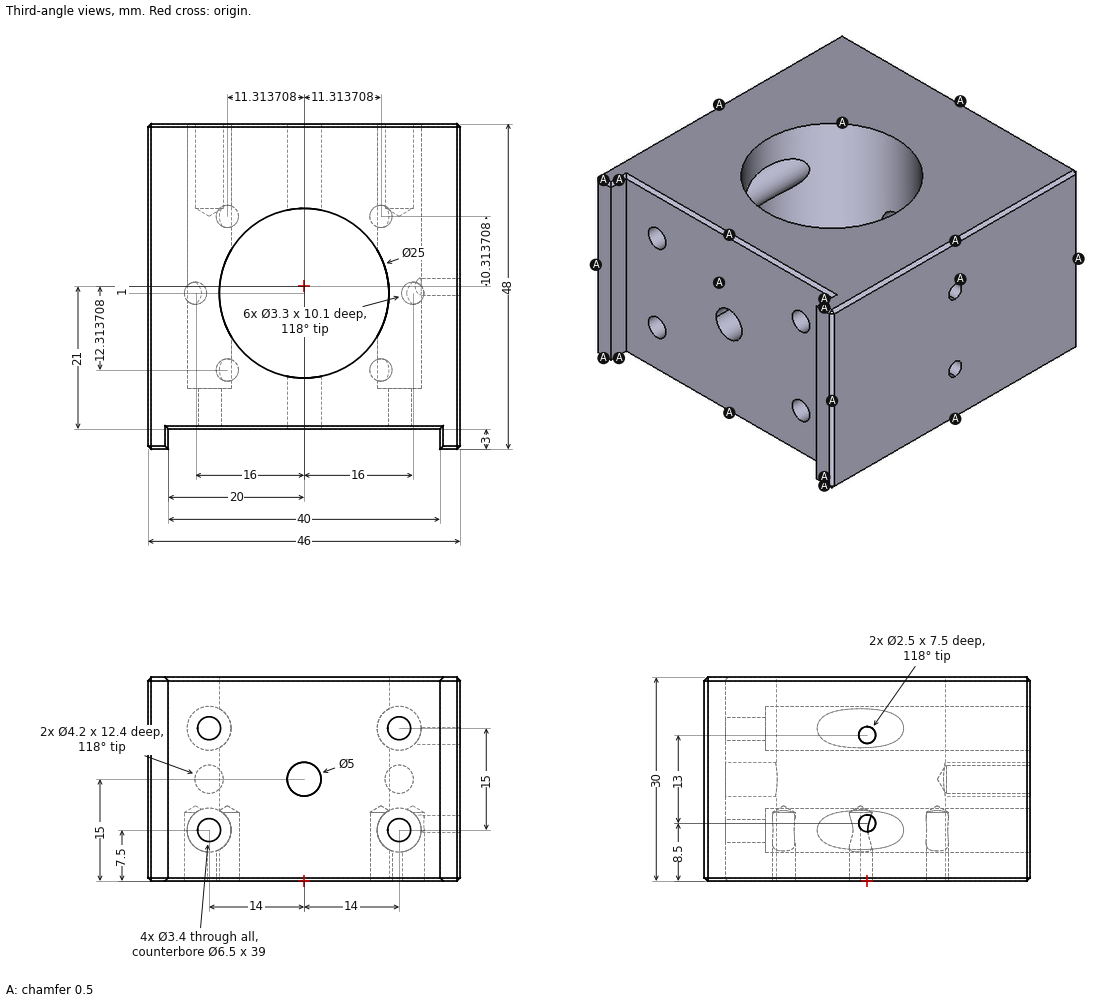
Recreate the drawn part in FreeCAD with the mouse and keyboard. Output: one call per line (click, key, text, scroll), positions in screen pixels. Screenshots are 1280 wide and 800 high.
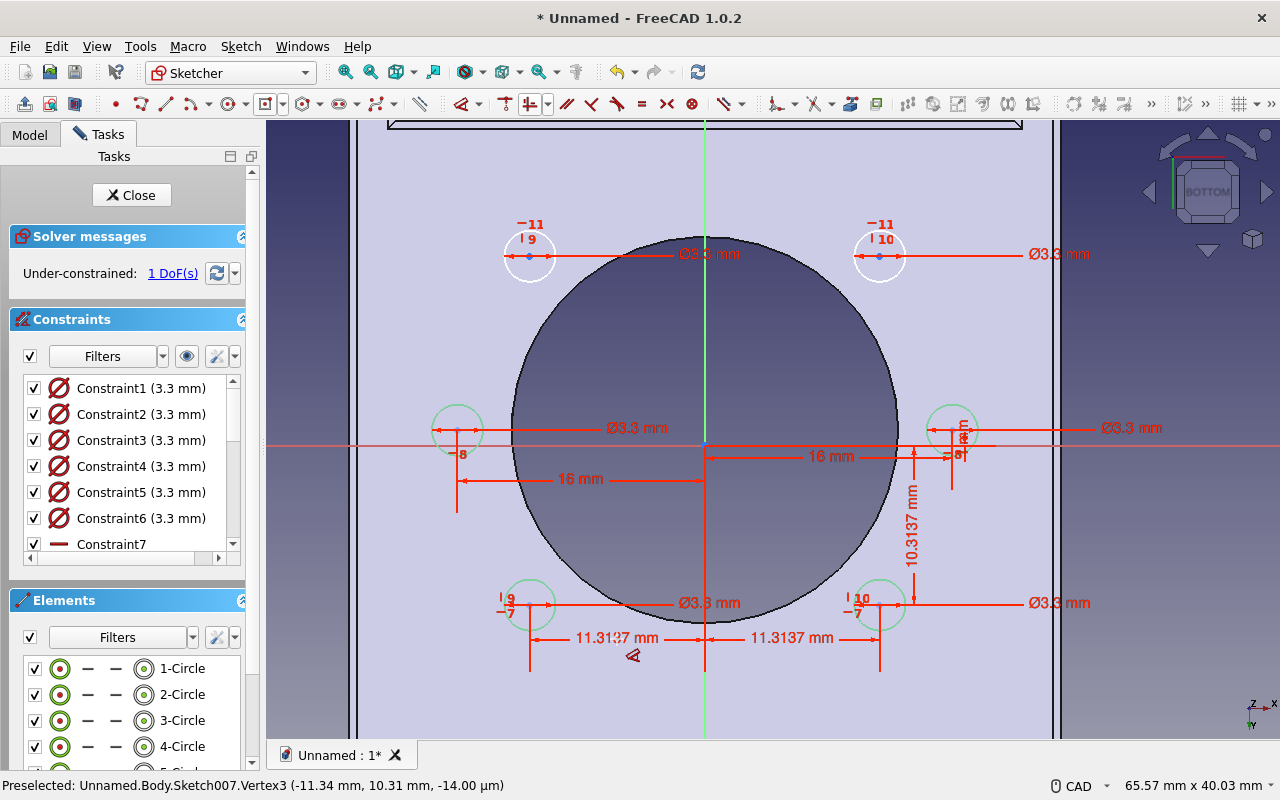
click(530, 256)
click(496, 351)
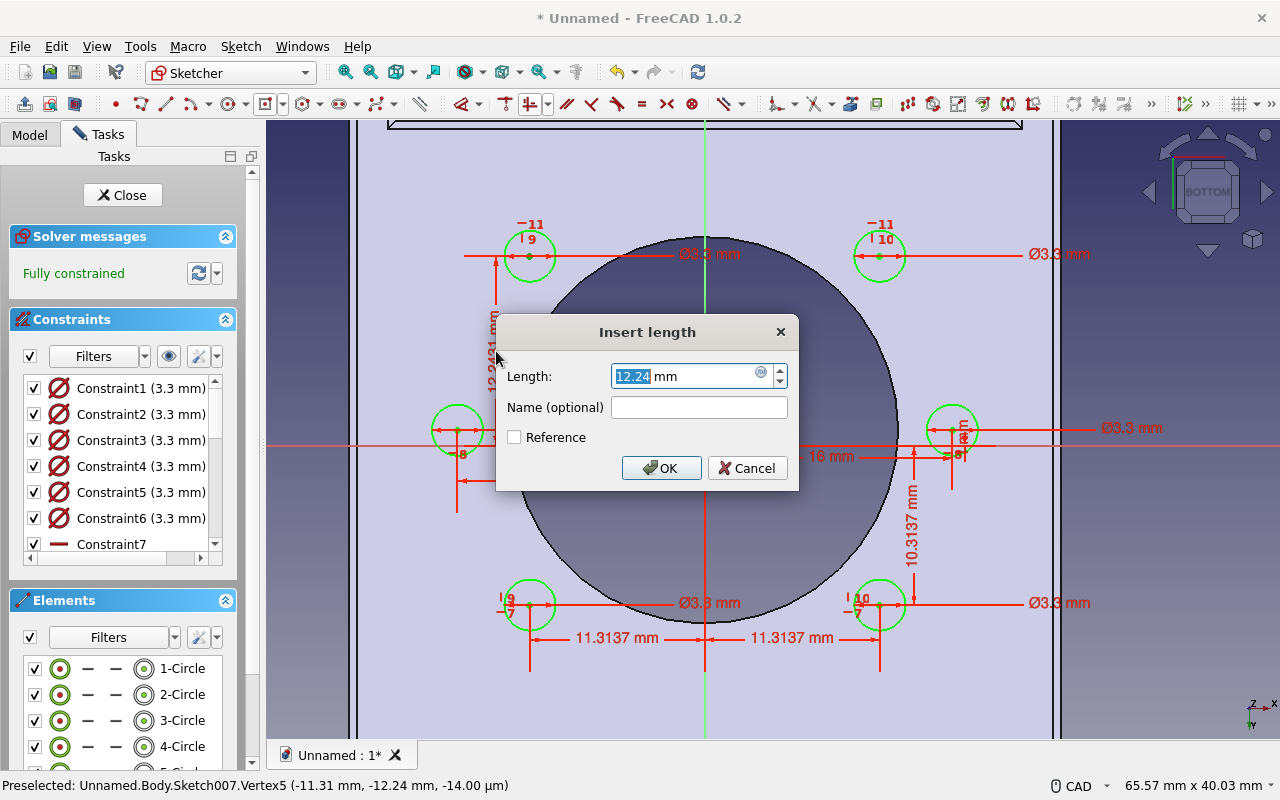
text(12.313708)
key(Return)
key(Escape)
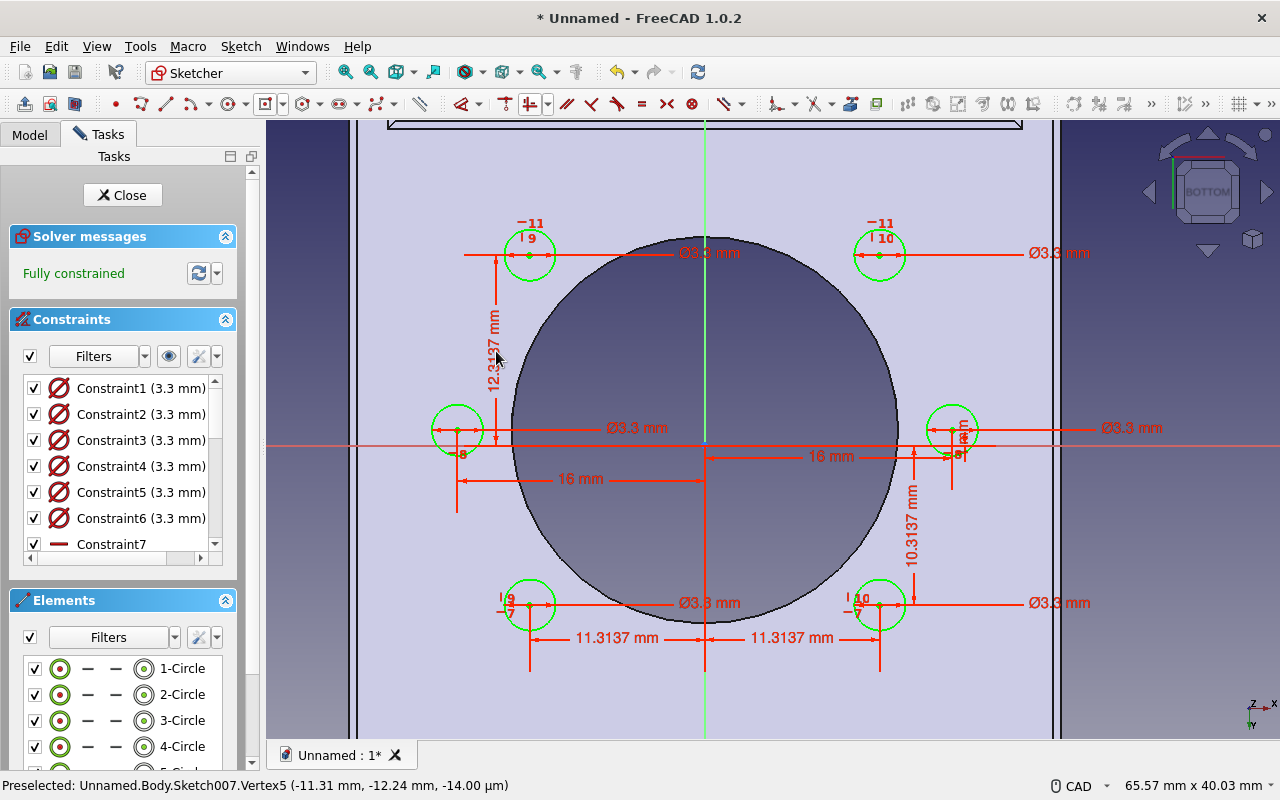
click(123, 195)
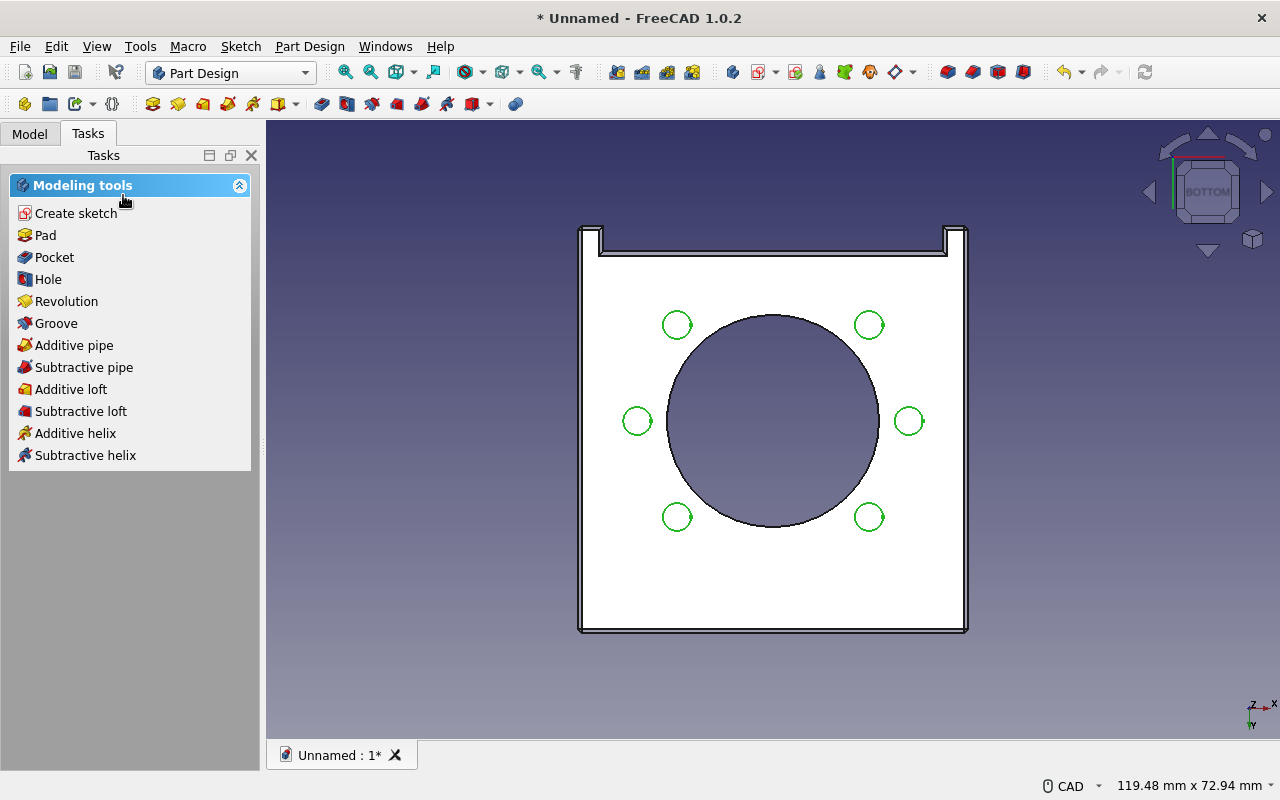
click(347, 104)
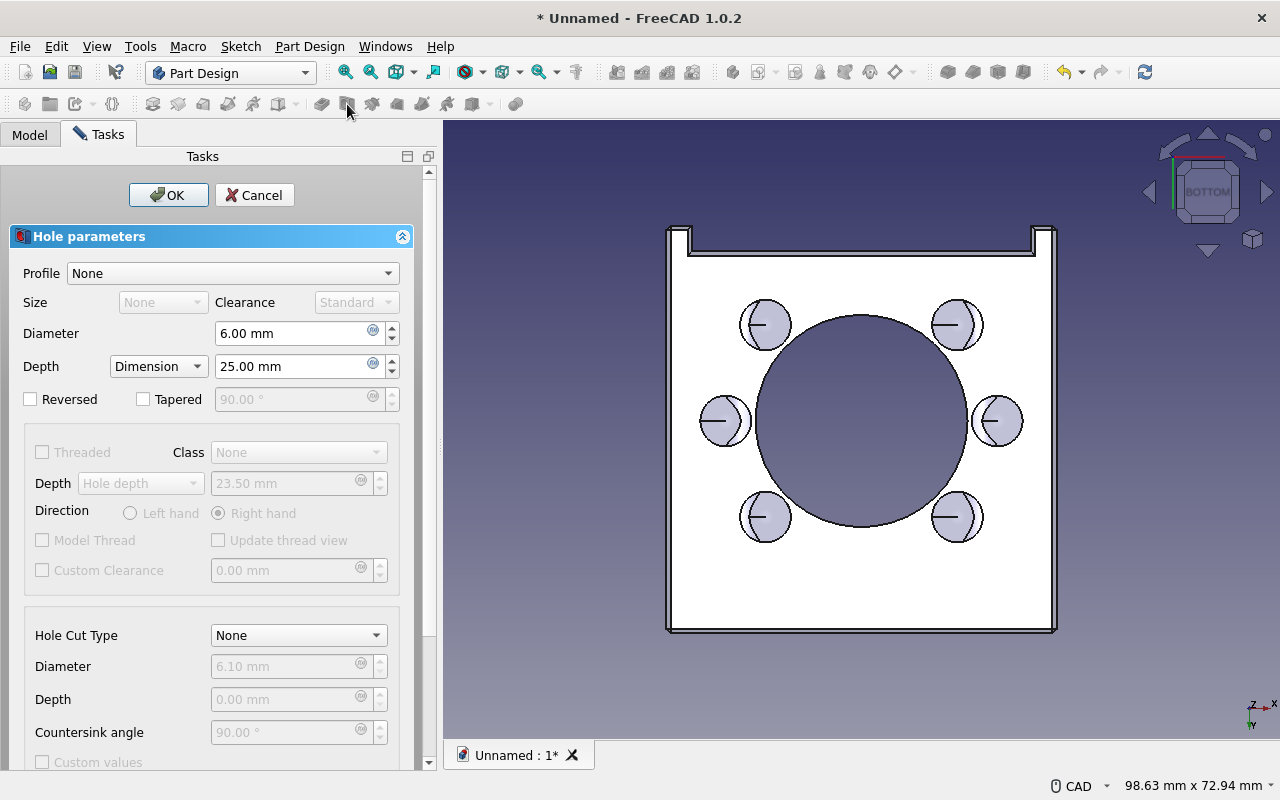
triple_click(300, 334)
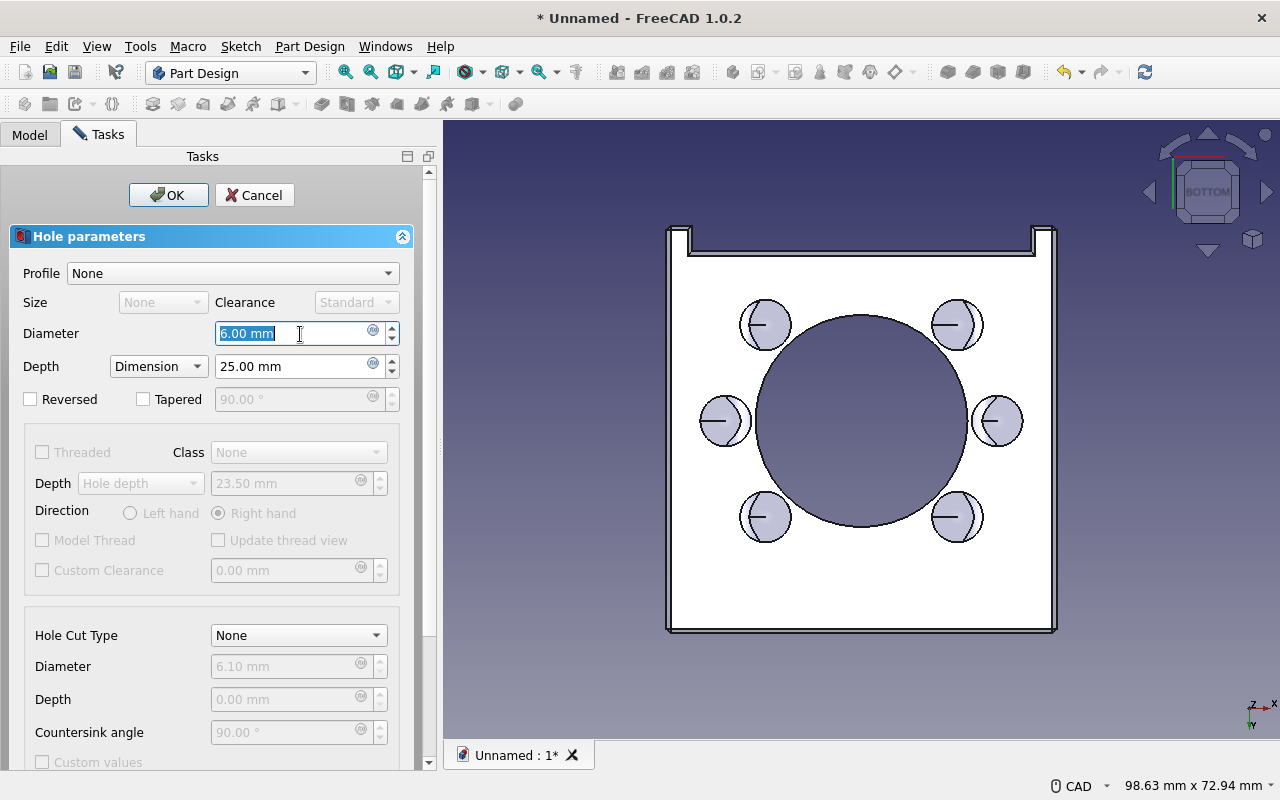
text(3.3)
key(Tab)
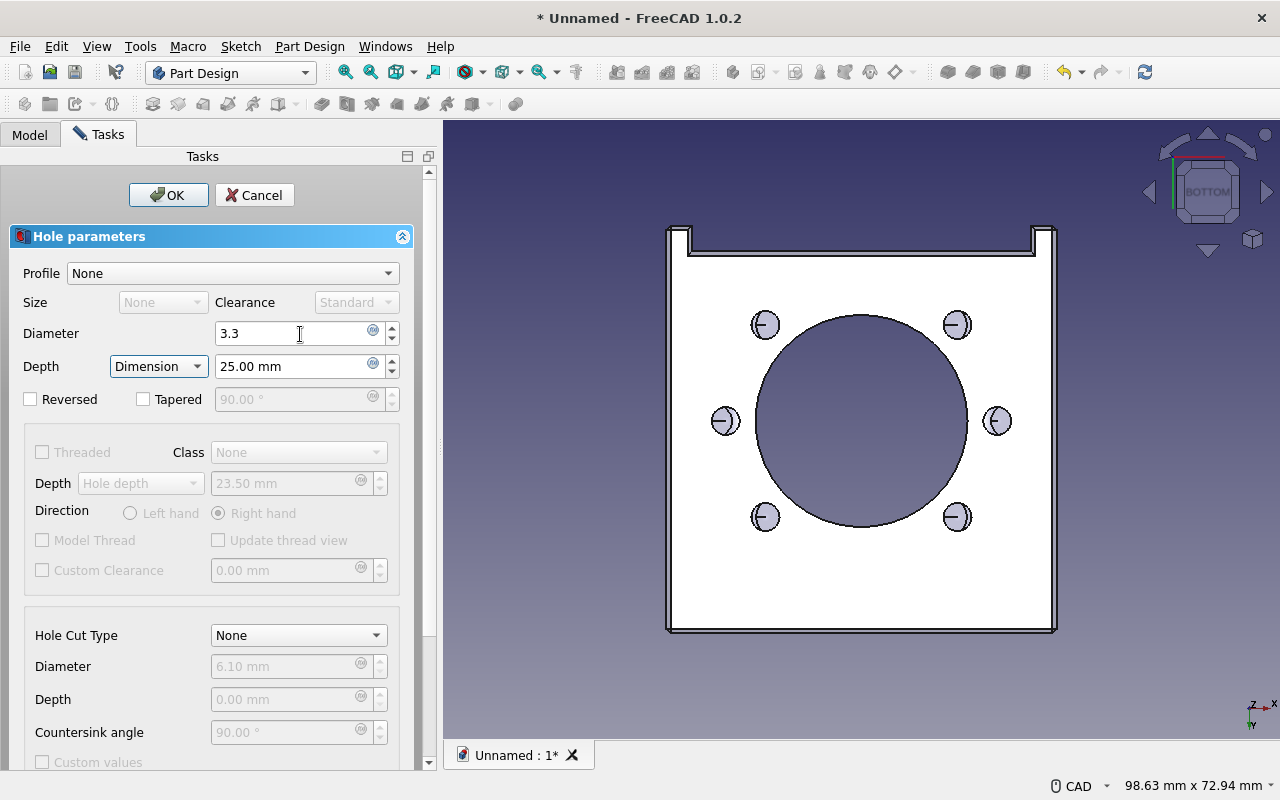
triple_click(300, 366)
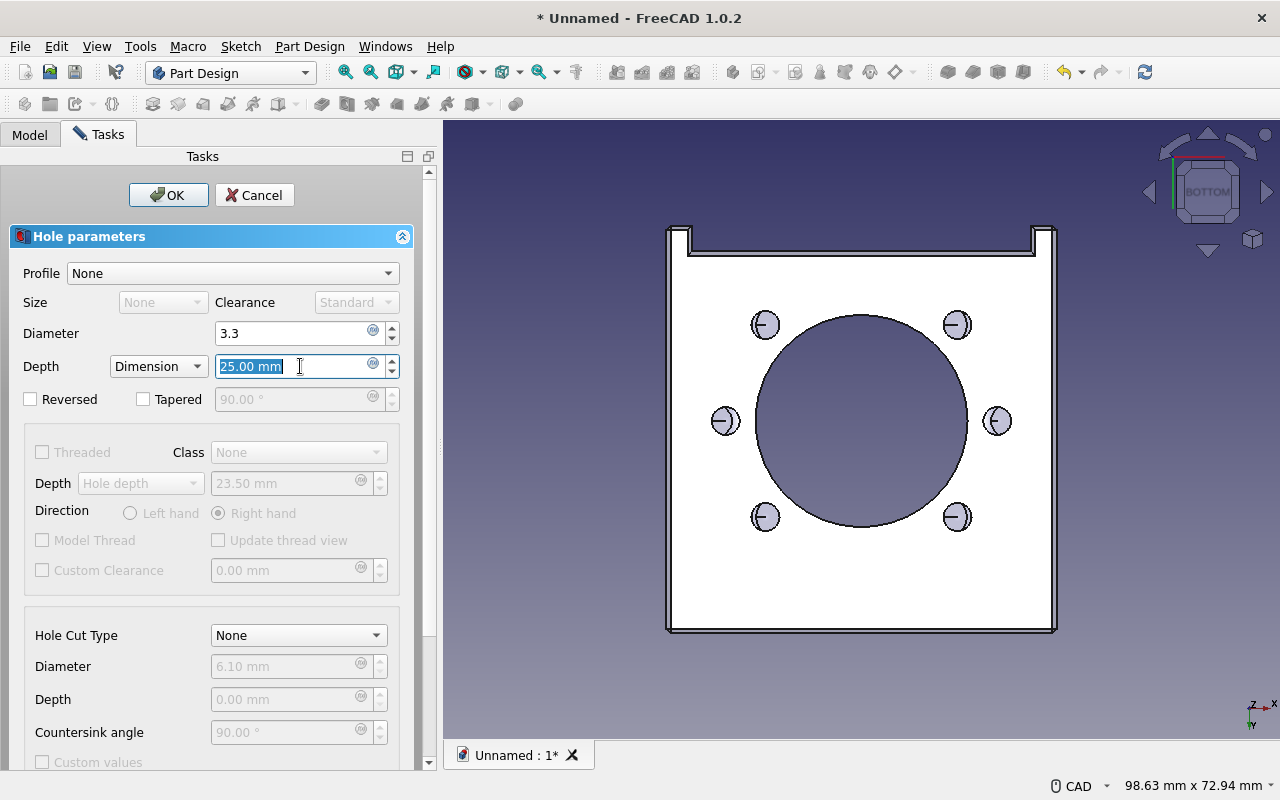
text(10.1)
key(Tab)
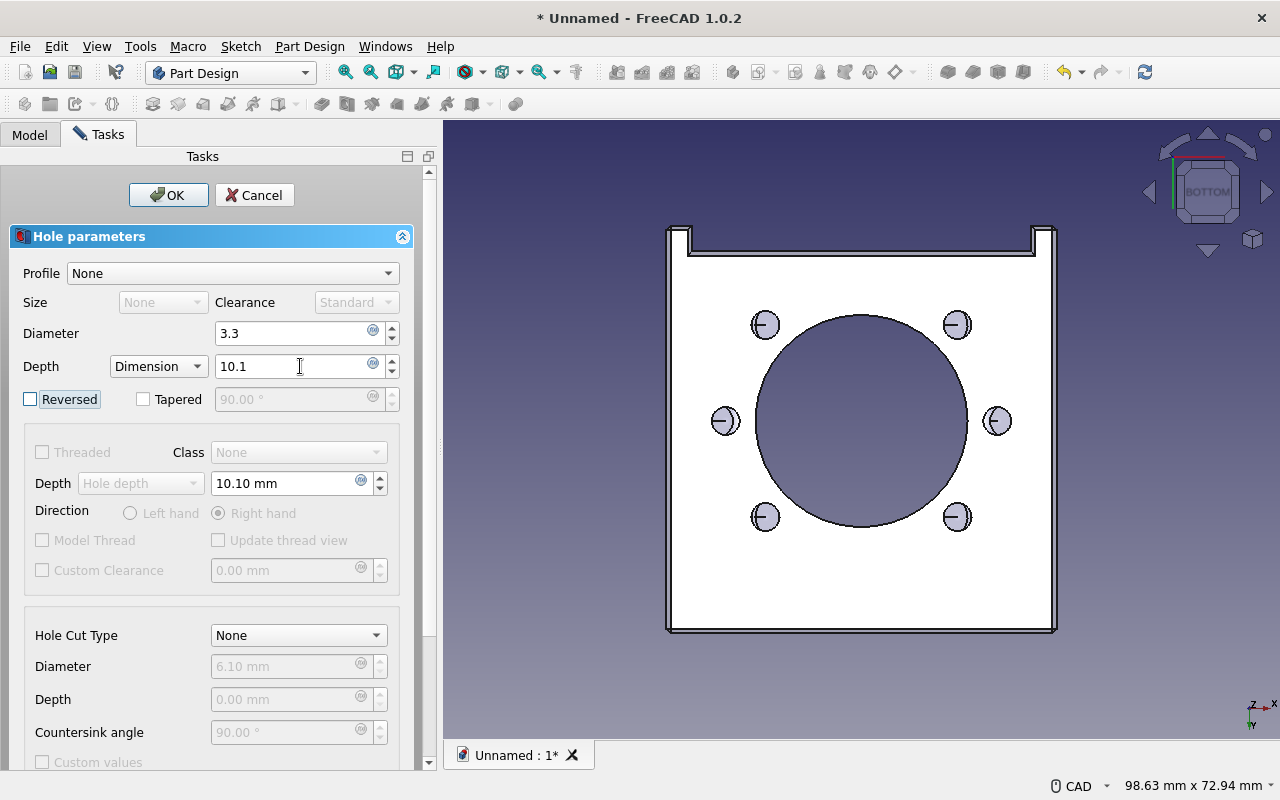
click(169, 195)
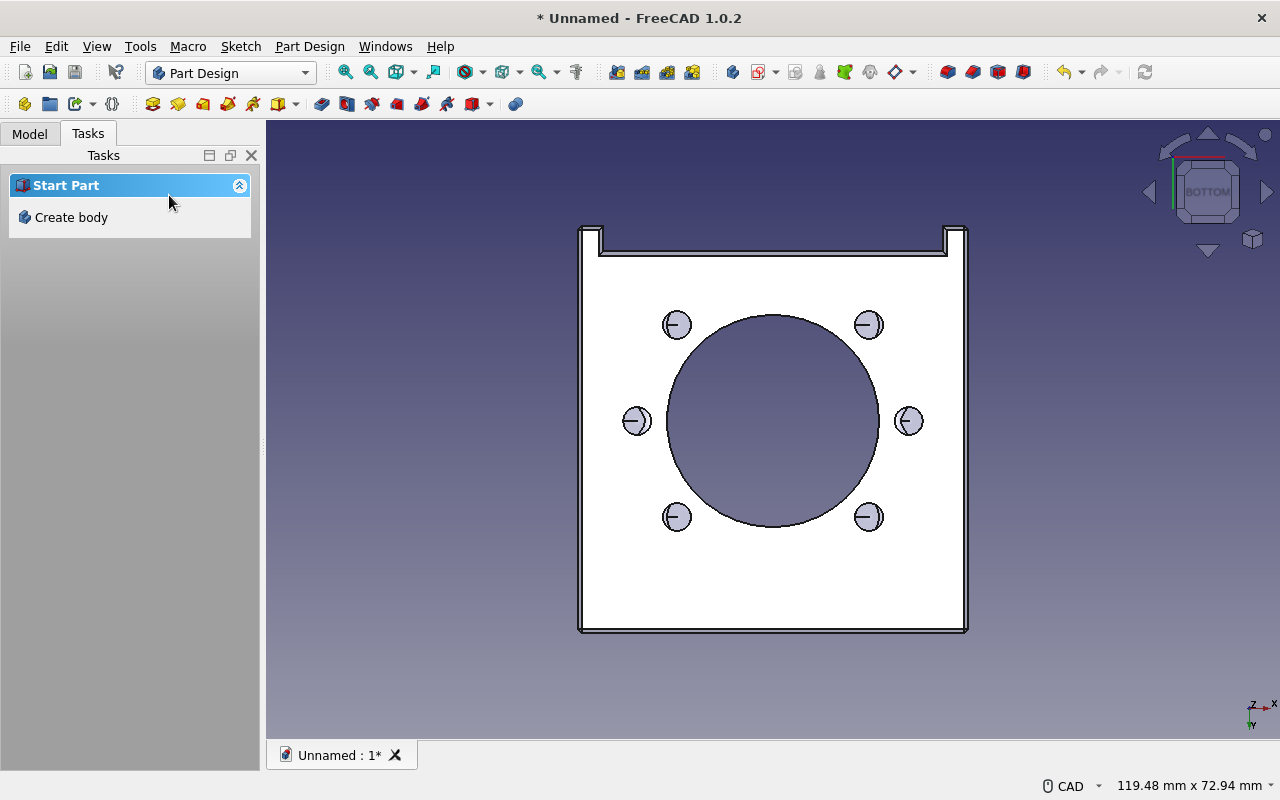
key(0)